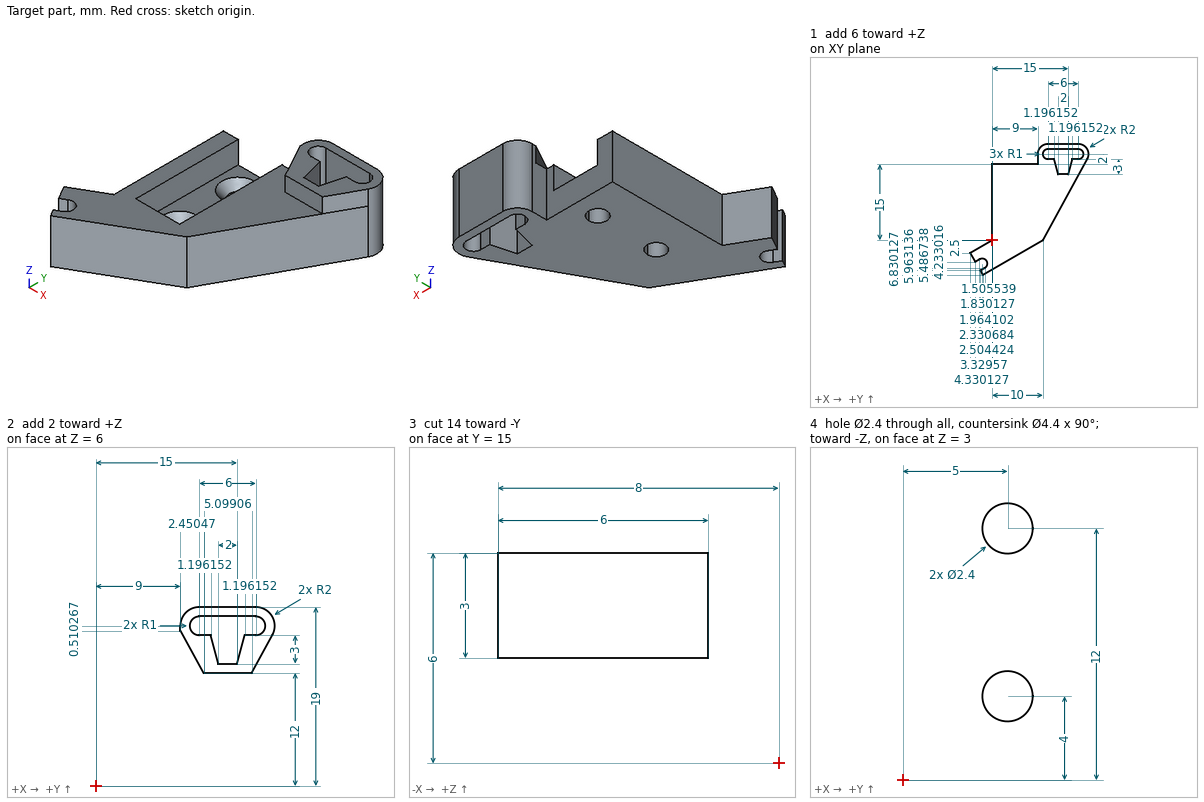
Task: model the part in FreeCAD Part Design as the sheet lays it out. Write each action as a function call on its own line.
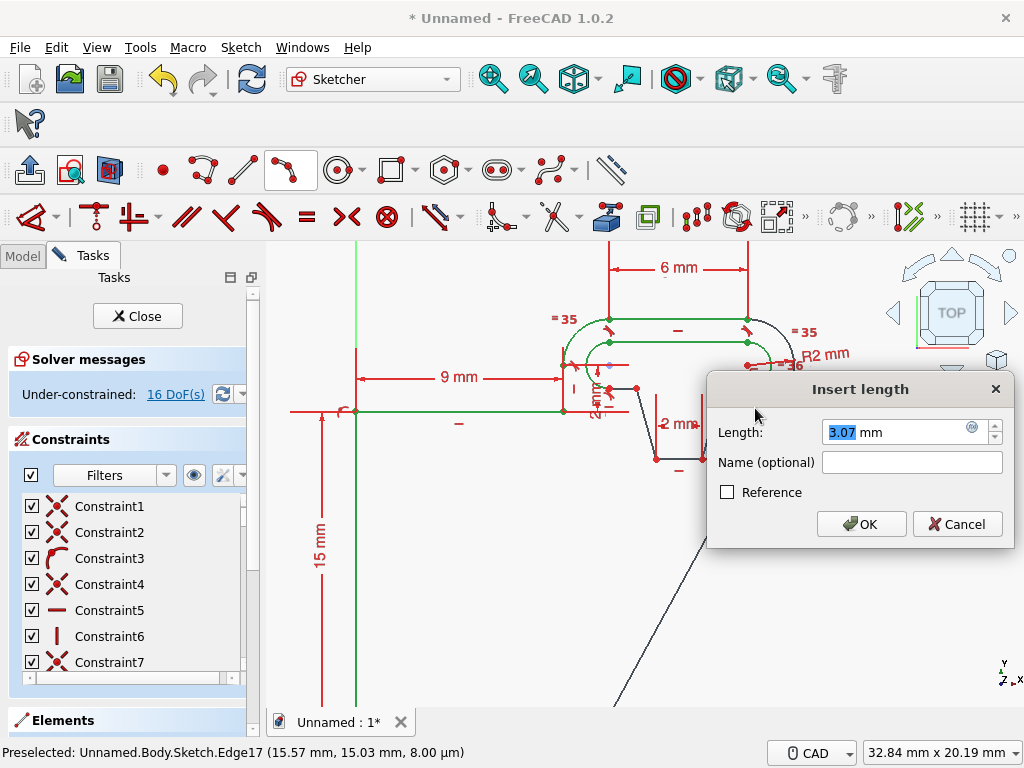
text(3)
key(Return)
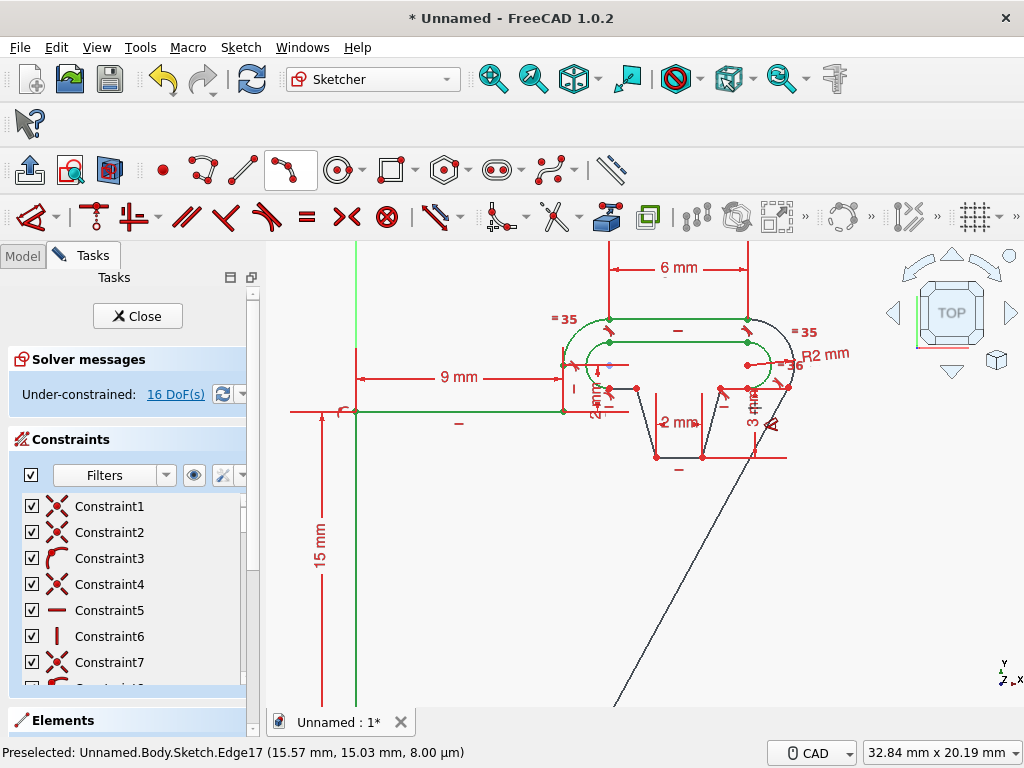
scroll(621, 357, down, 4)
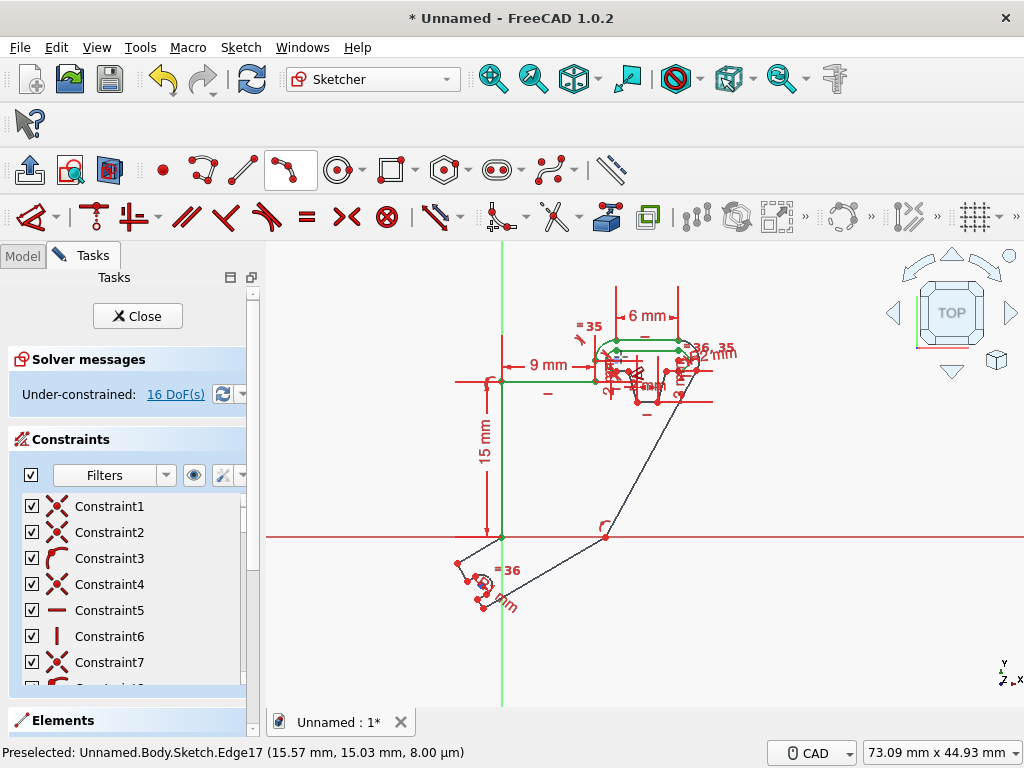
click(606, 537)
click(578, 571)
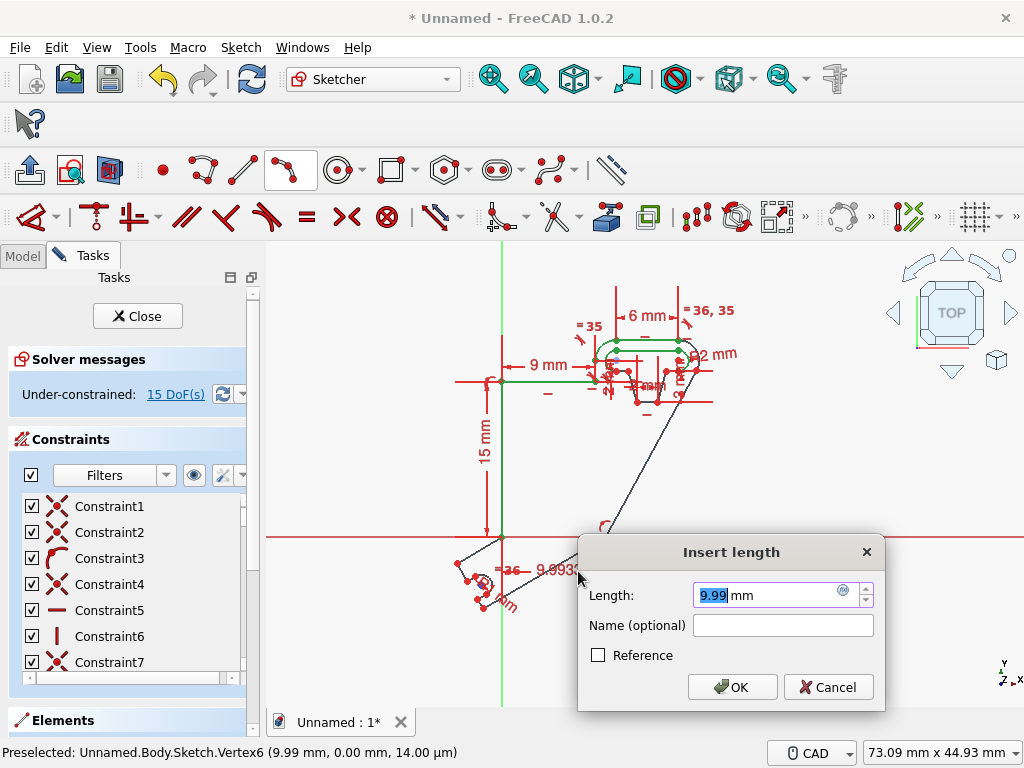
text(10)
key(Return)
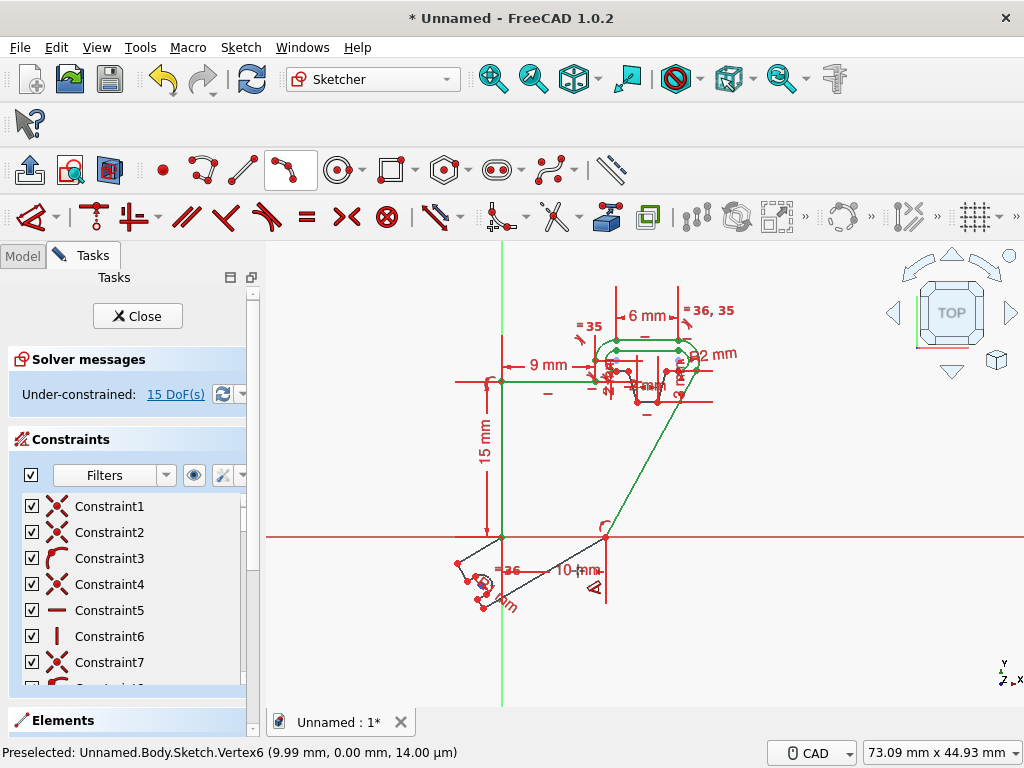
click(658, 402)
click(580, 344)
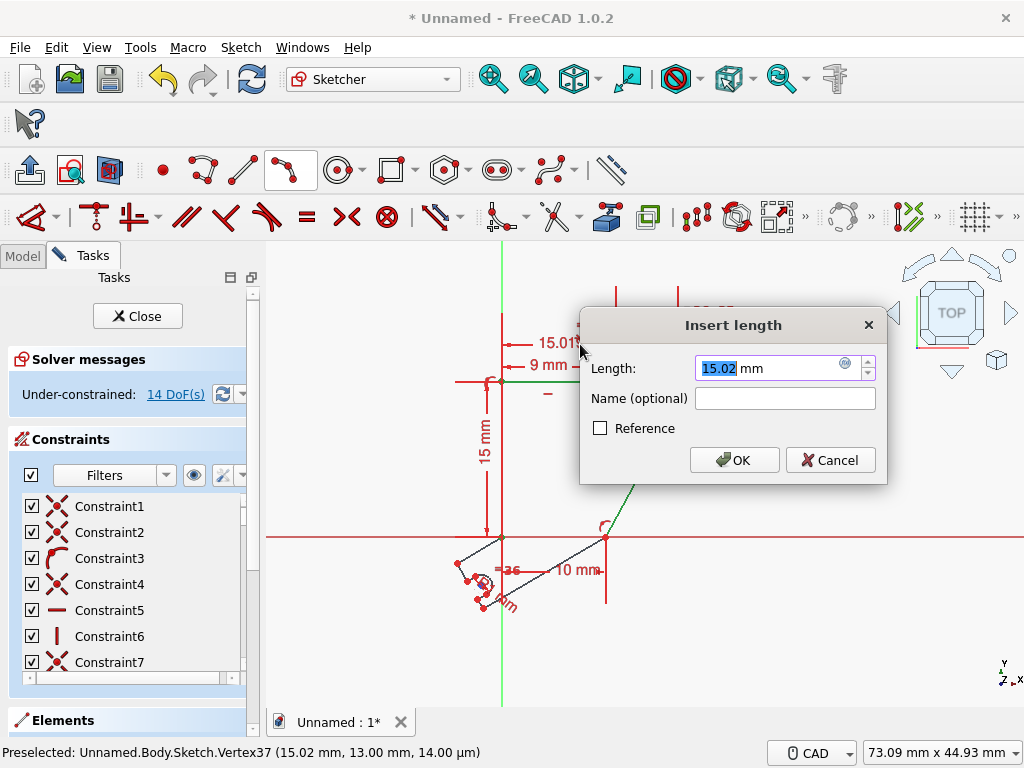
text(15)
key(Return)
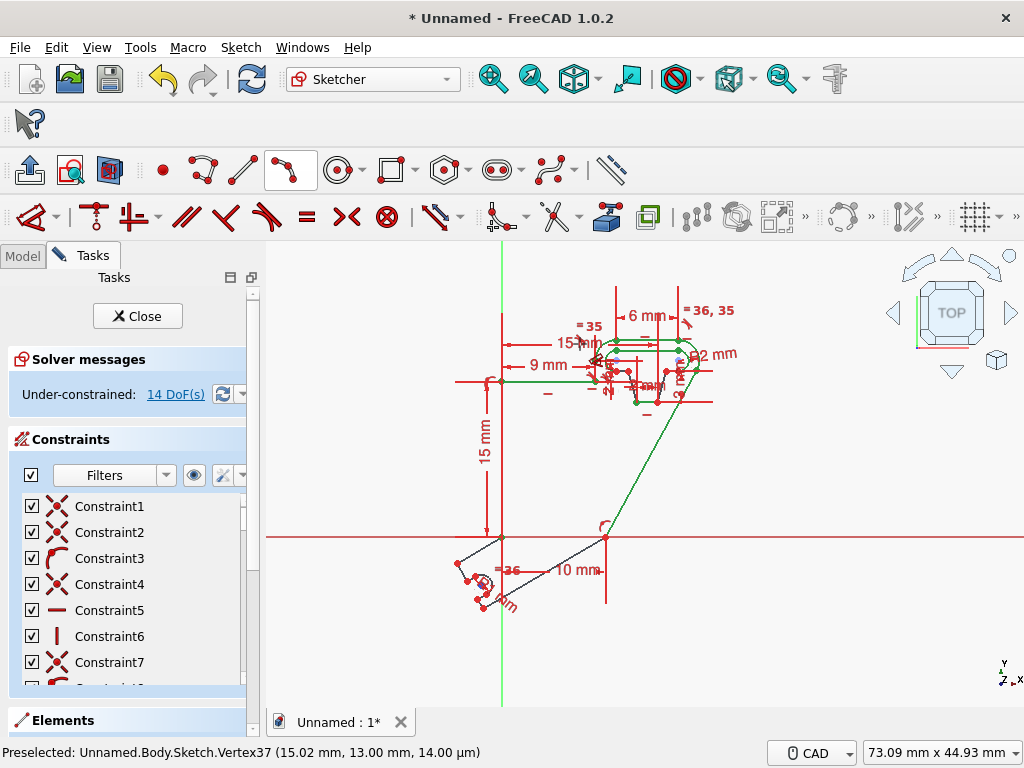
scroll(457, 564, up, 3)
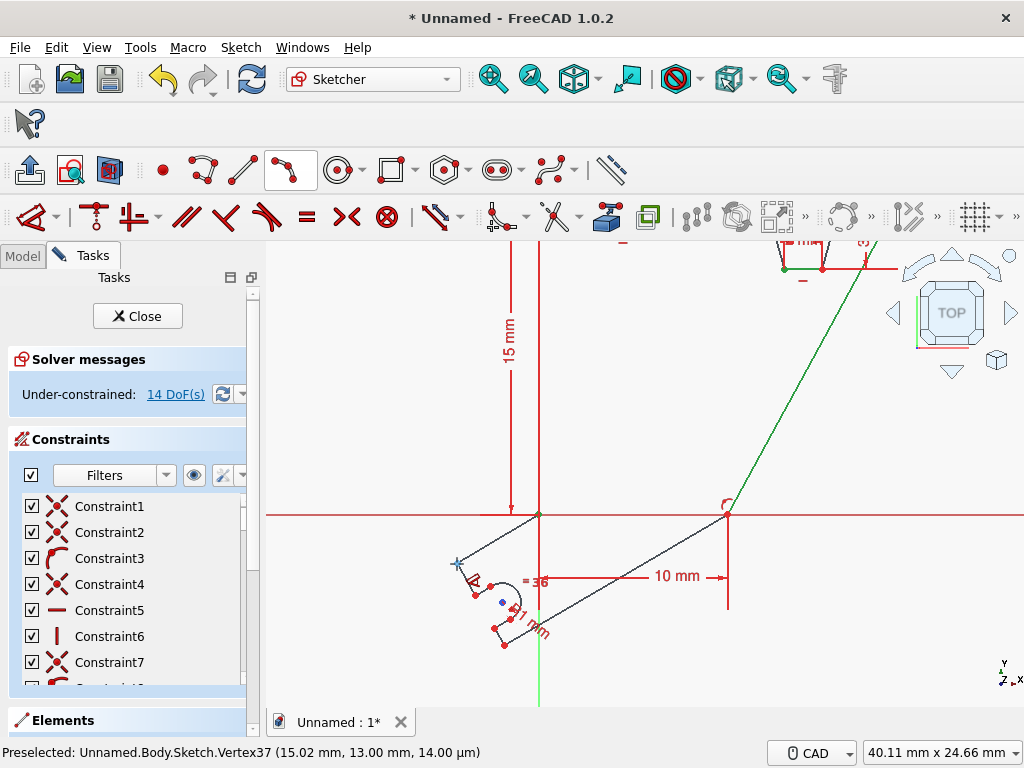
click(457, 563)
click(423, 539)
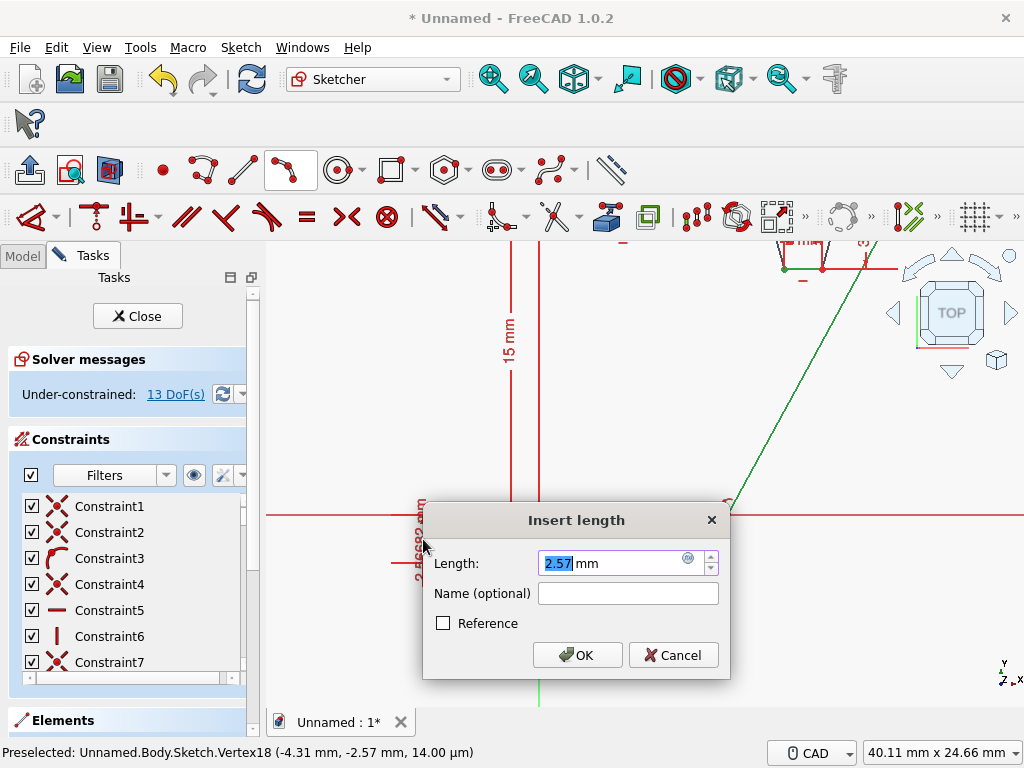
text(2.5)
key(Return)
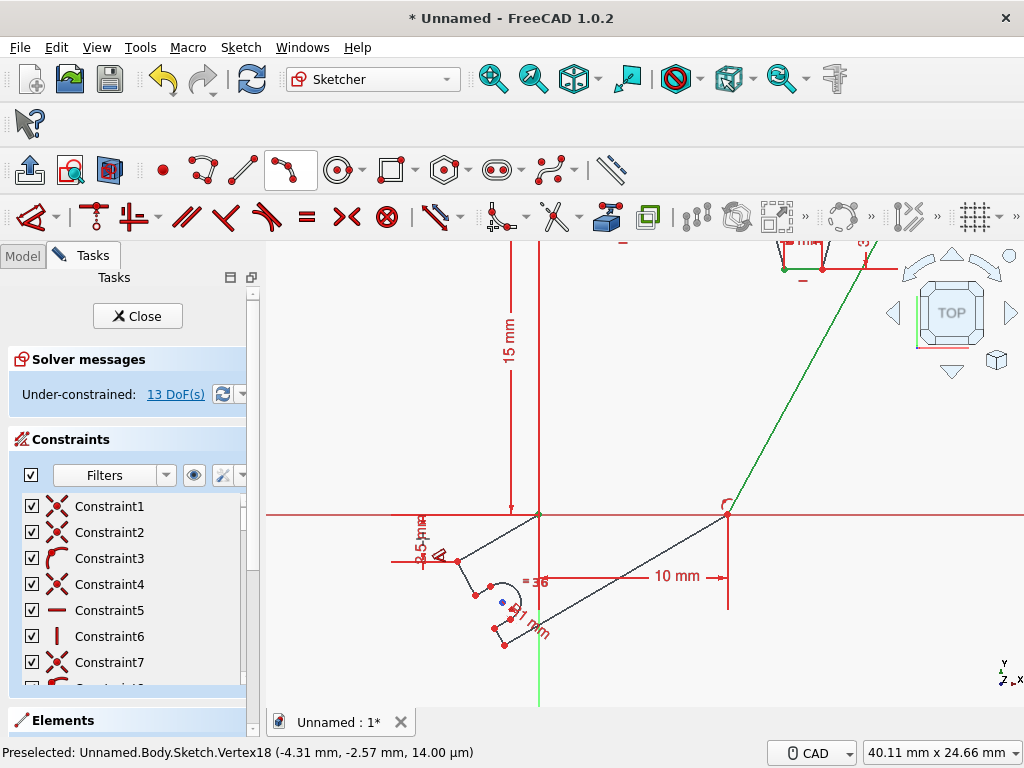
scroll(457, 564, down, 3)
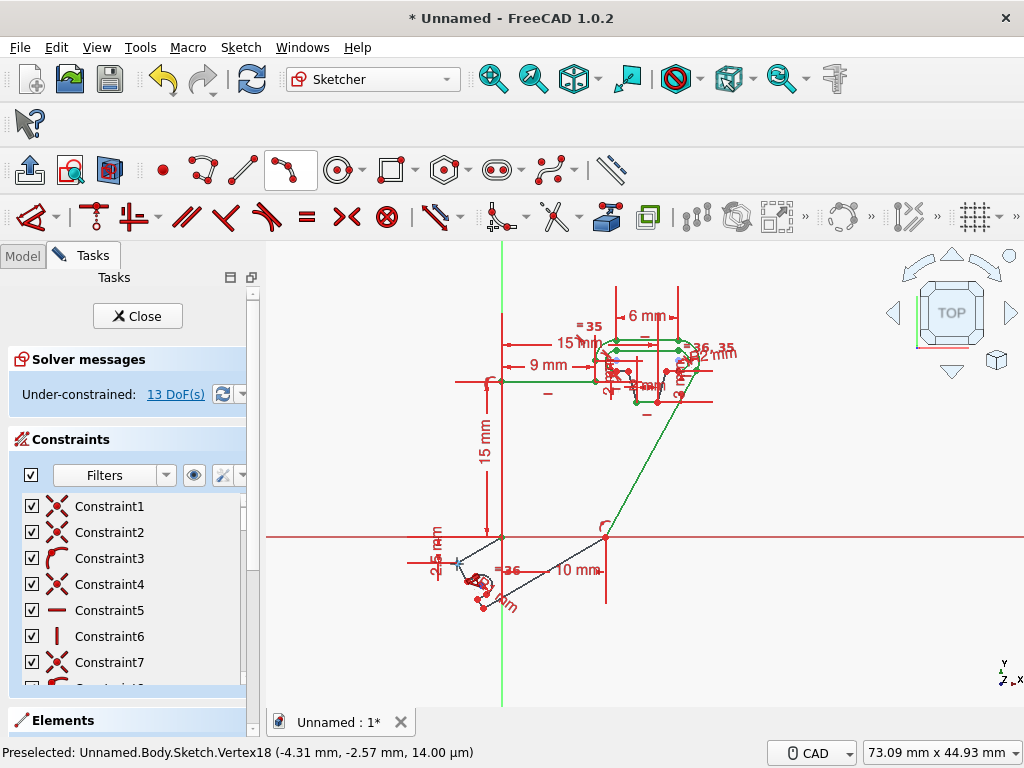
scroll(672, 371, up, 6)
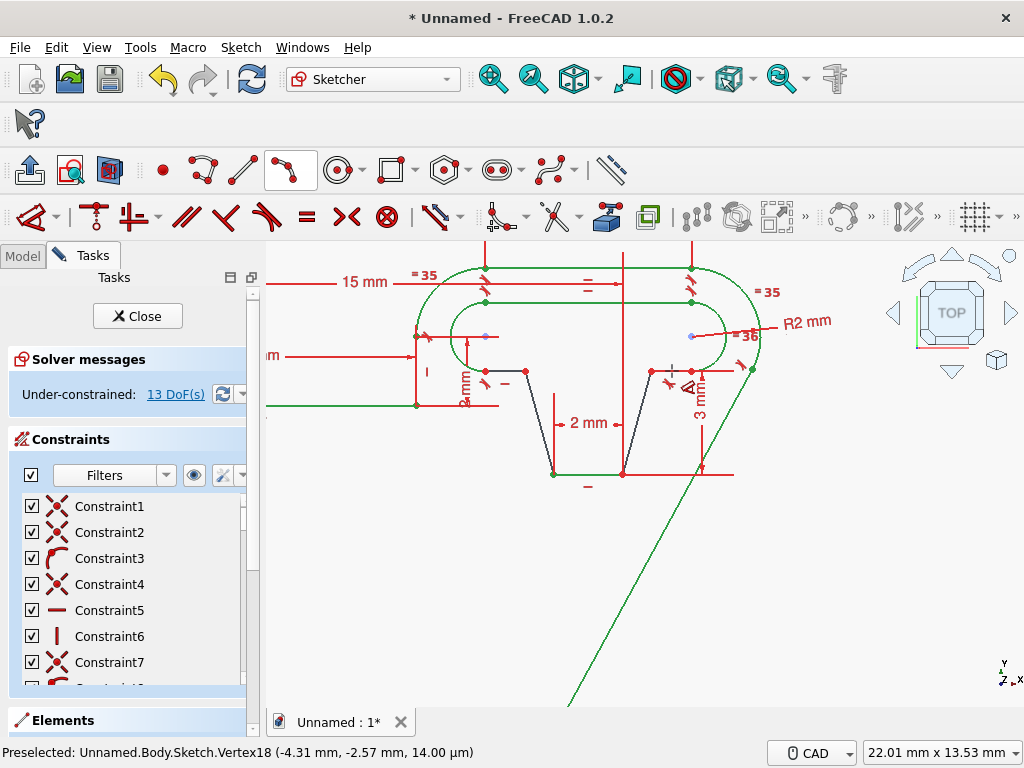
click(671, 371)
click(671, 337)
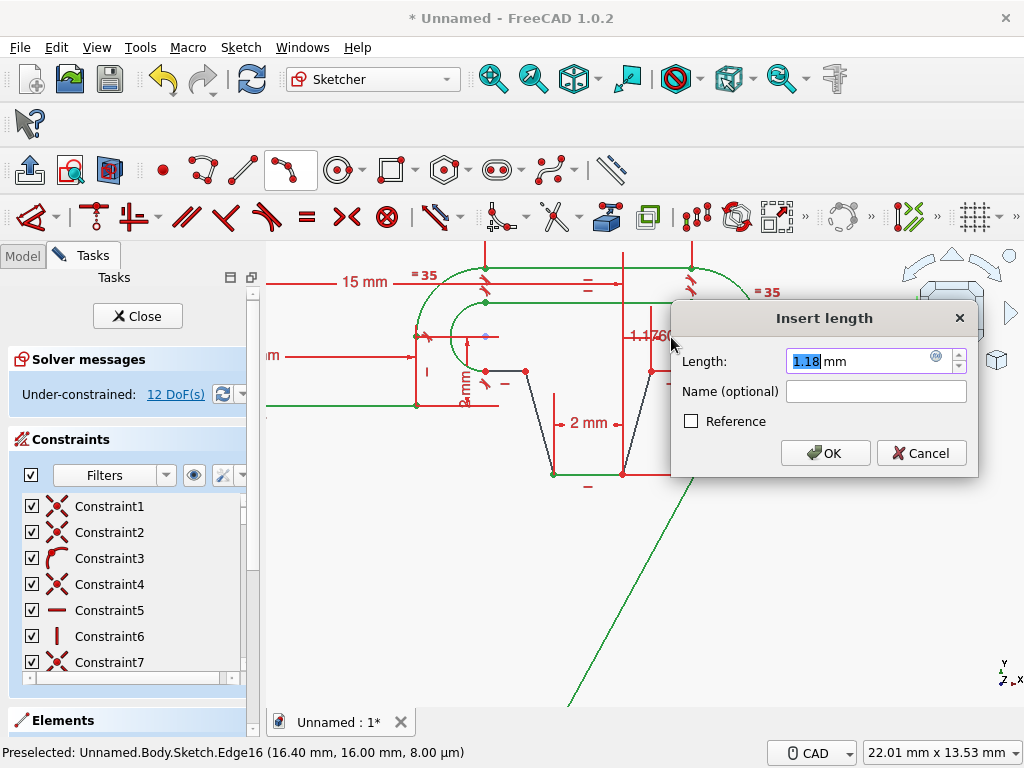
text(1.196152)
key(Return)